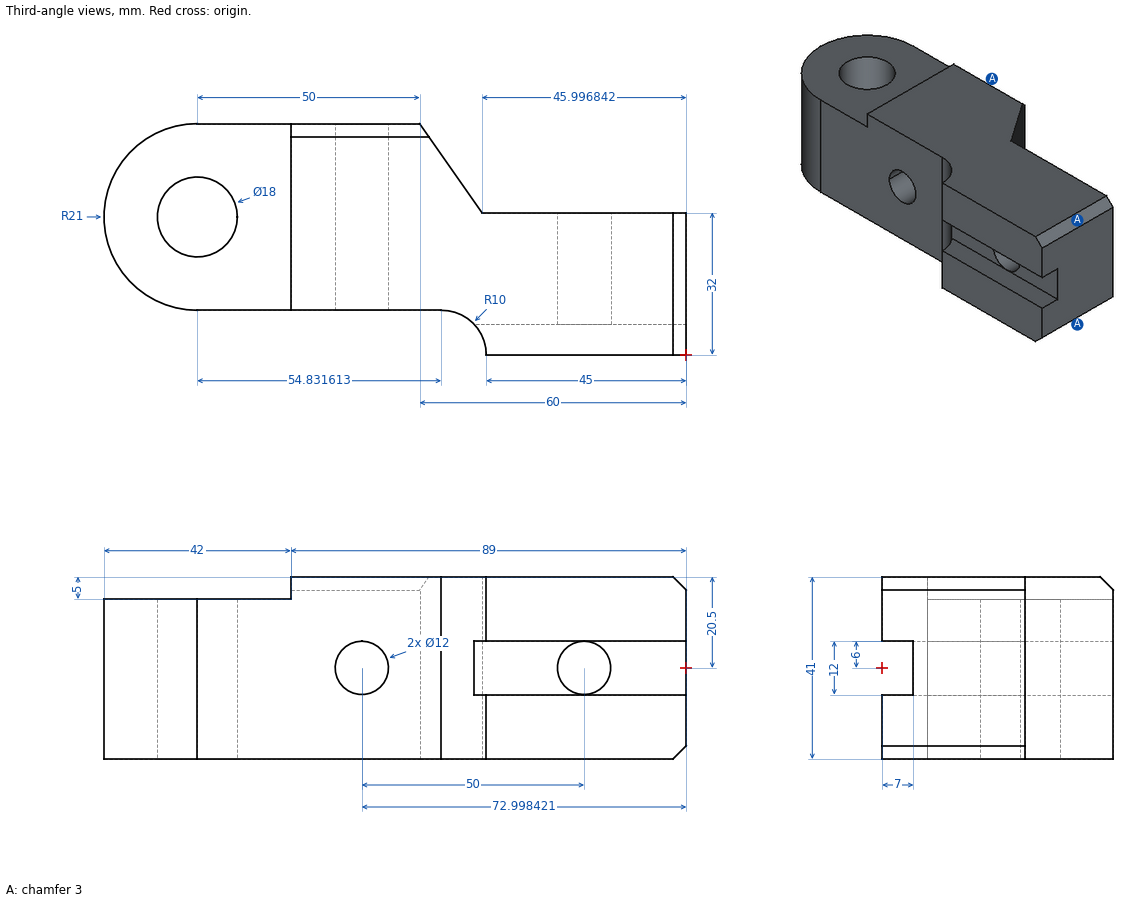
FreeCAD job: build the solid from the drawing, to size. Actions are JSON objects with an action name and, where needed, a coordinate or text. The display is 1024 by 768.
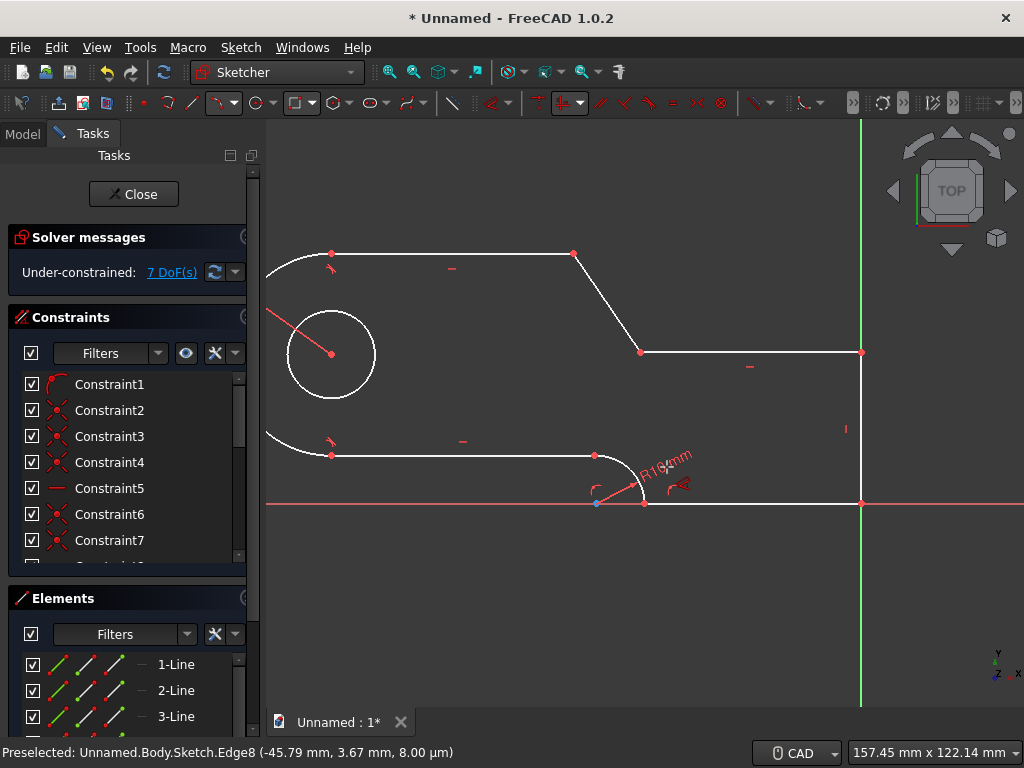
{"action": "left_click", "coordinate": [362, 324]}
{"action": "left_click", "coordinate": [385, 301]}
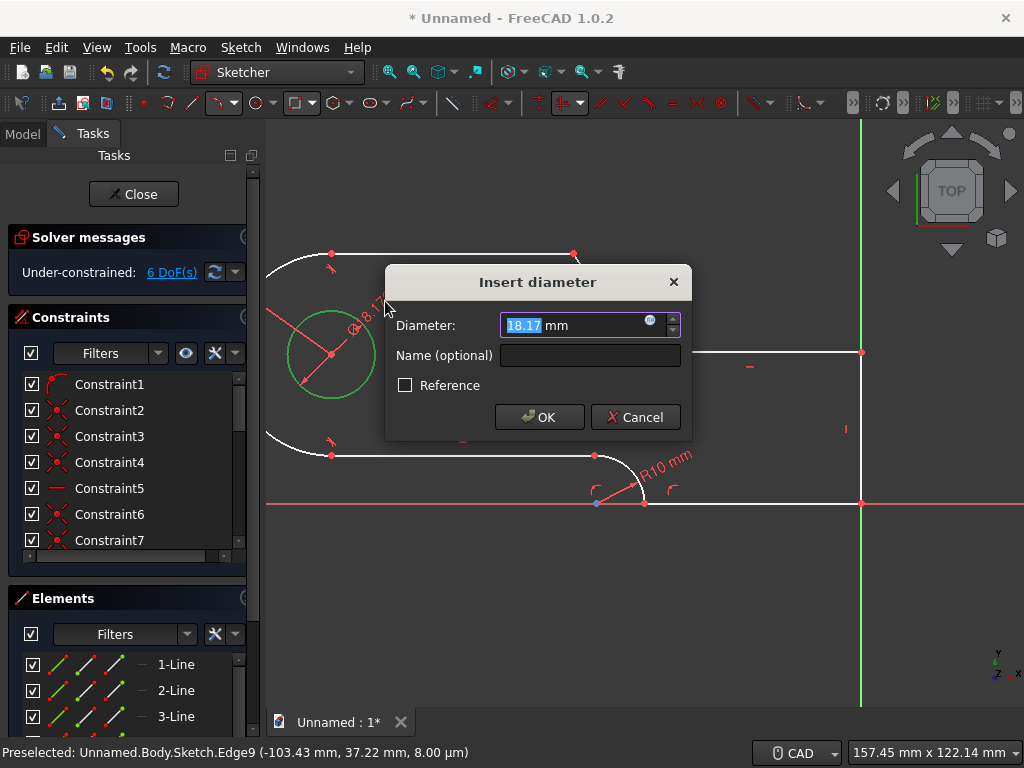
{"action": "type", "text": "18"}
{"action": "key", "text": "Return"}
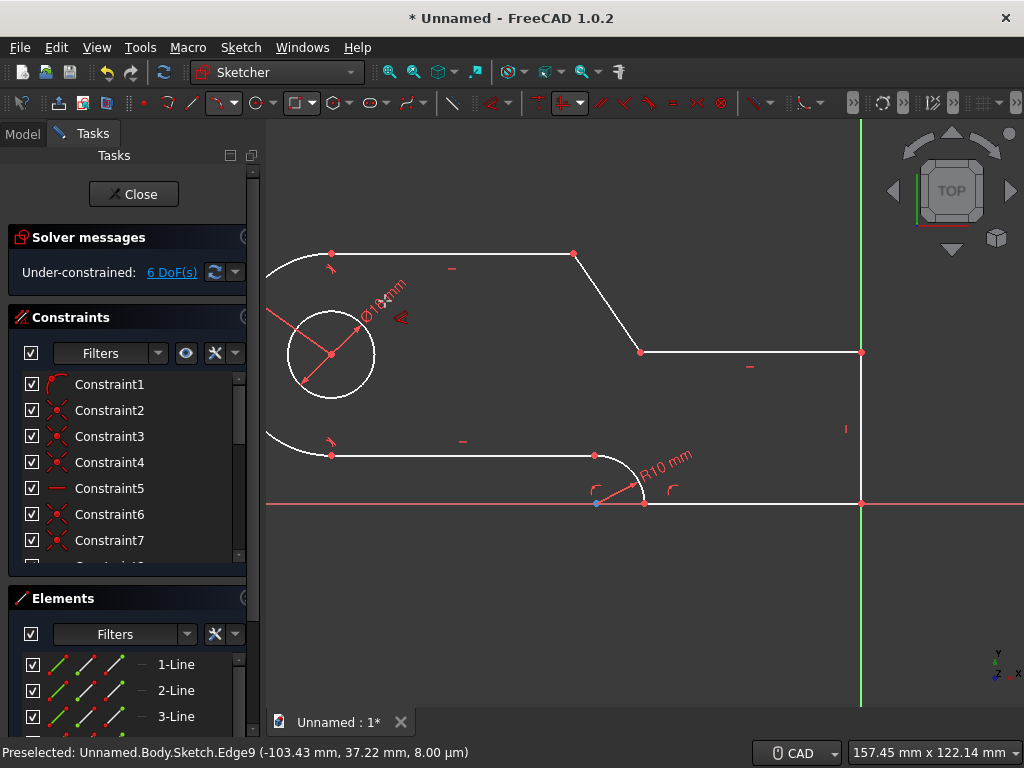
{"action": "left_click", "coordinate": [709, 504]}
{"action": "left_click", "coordinate": [752, 538]}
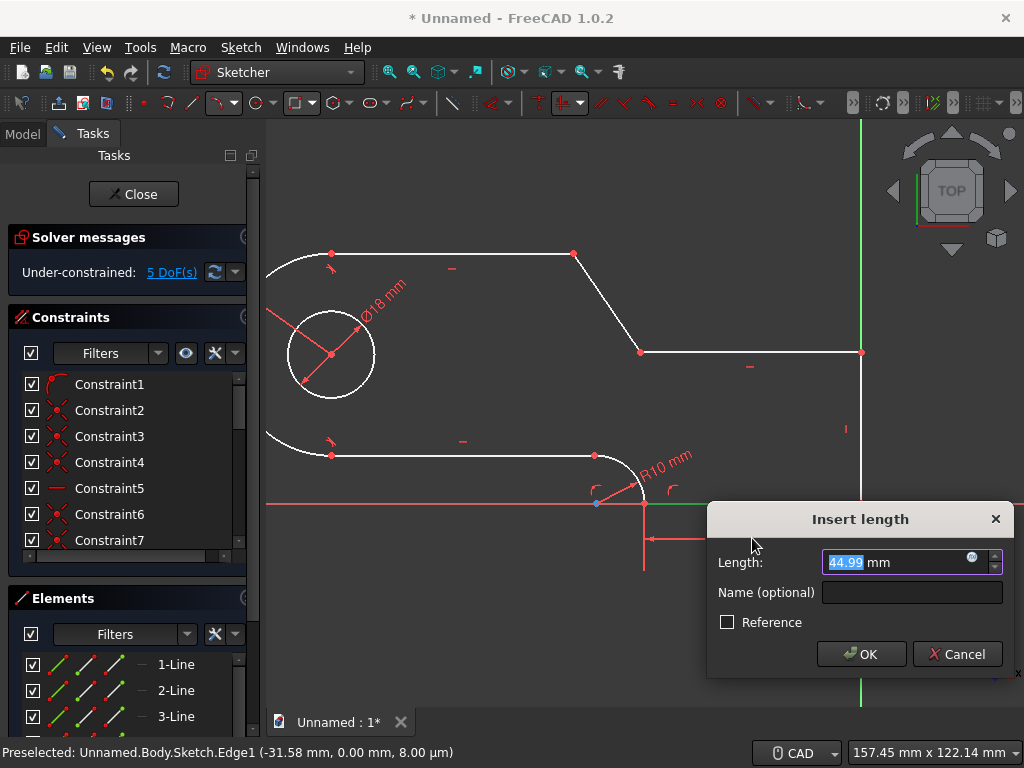
{"action": "type", "text": "45"}
{"action": "key", "text": "Return"}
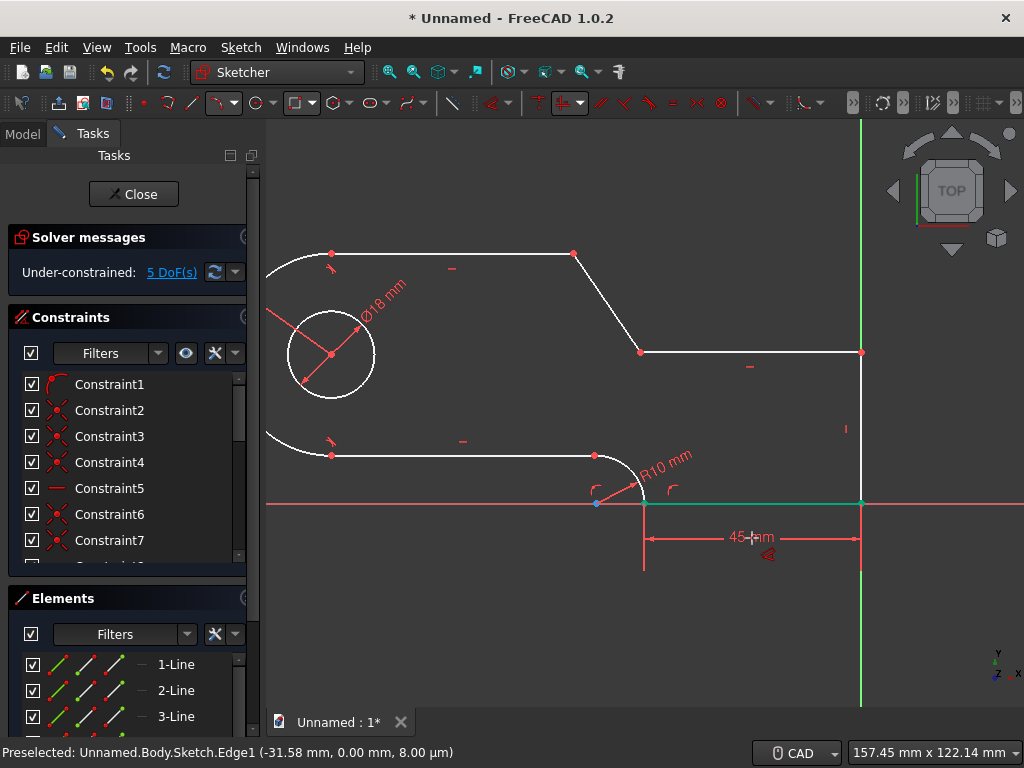
{"action": "scroll", "coordinate": [639, 483], "scroll_direction": "down", "scroll_amount": 2}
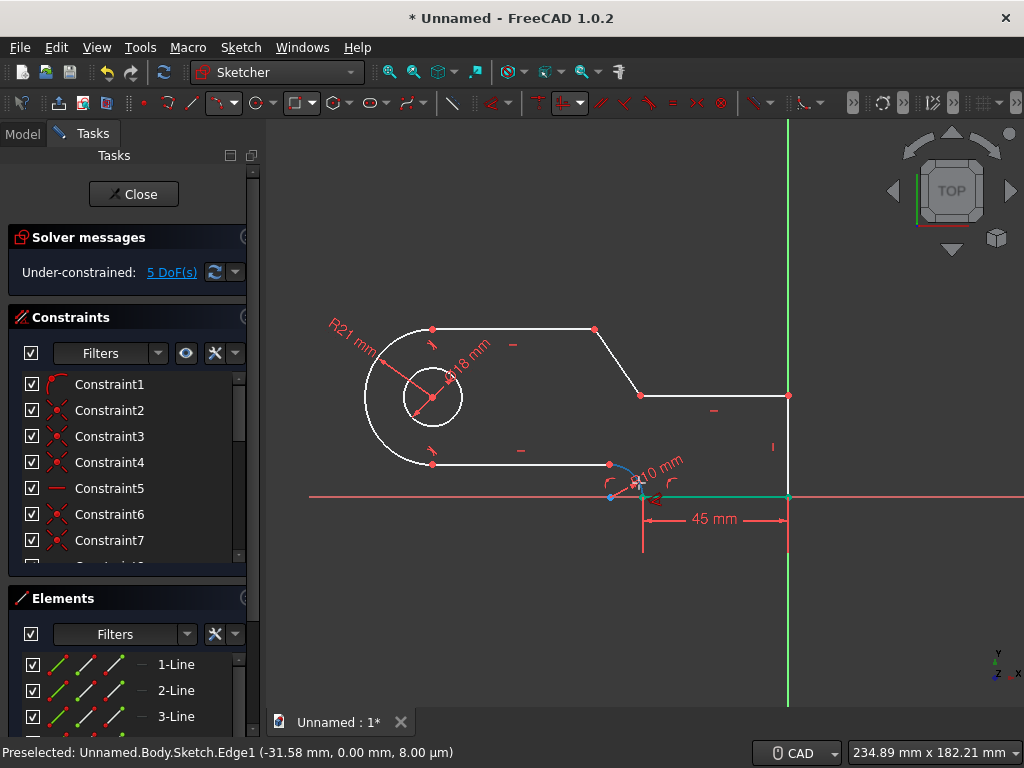
{"action": "left_click", "coordinate": [788, 467]}
{"action": "left_click", "coordinate": [822, 446]}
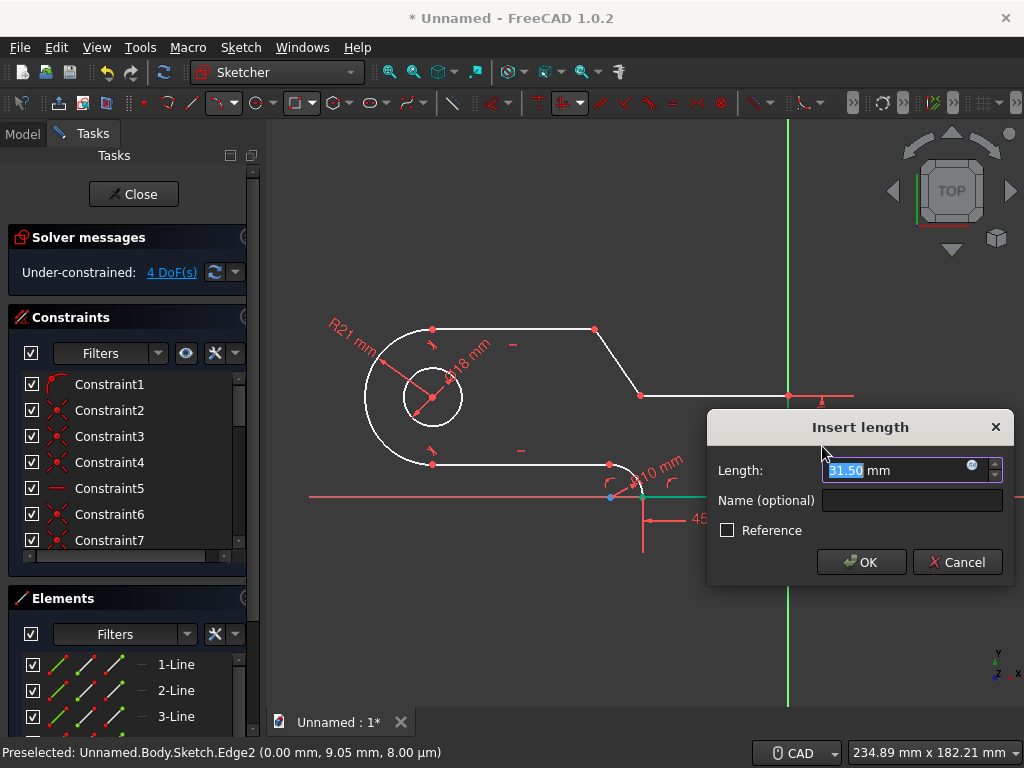
{"action": "type", "text": "32"}
{"action": "key", "text": "Return"}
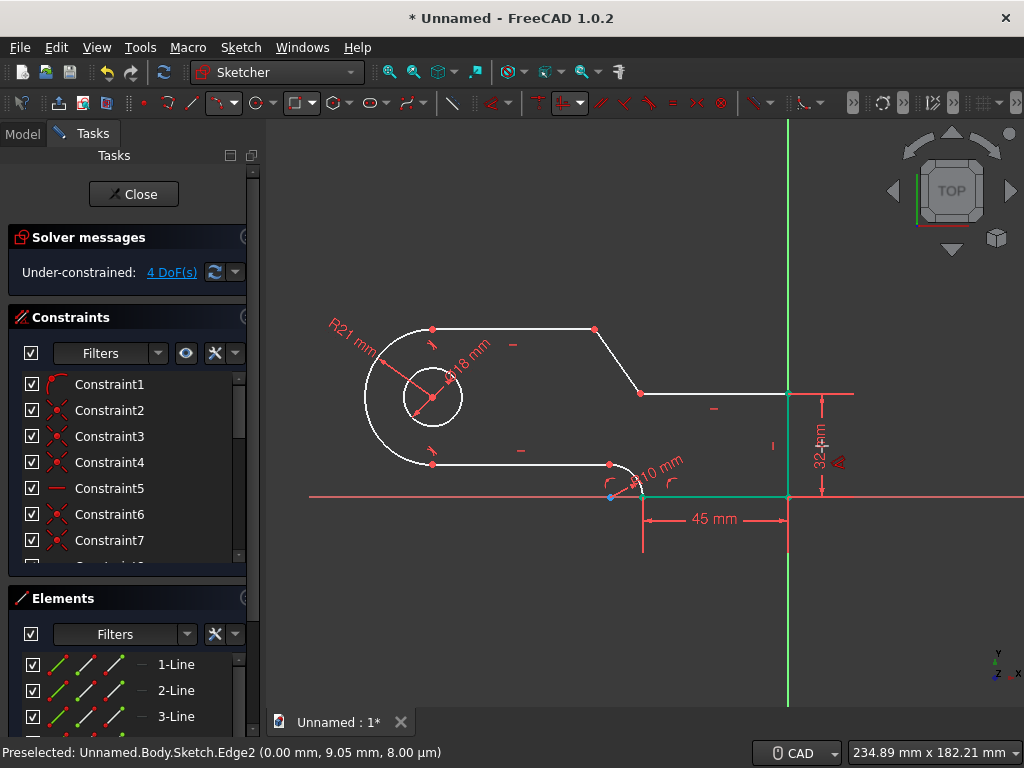
{"action": "left_click", "coordinate": [546, 329]}
{"action": "left_click", "coordinate": [514, 295]}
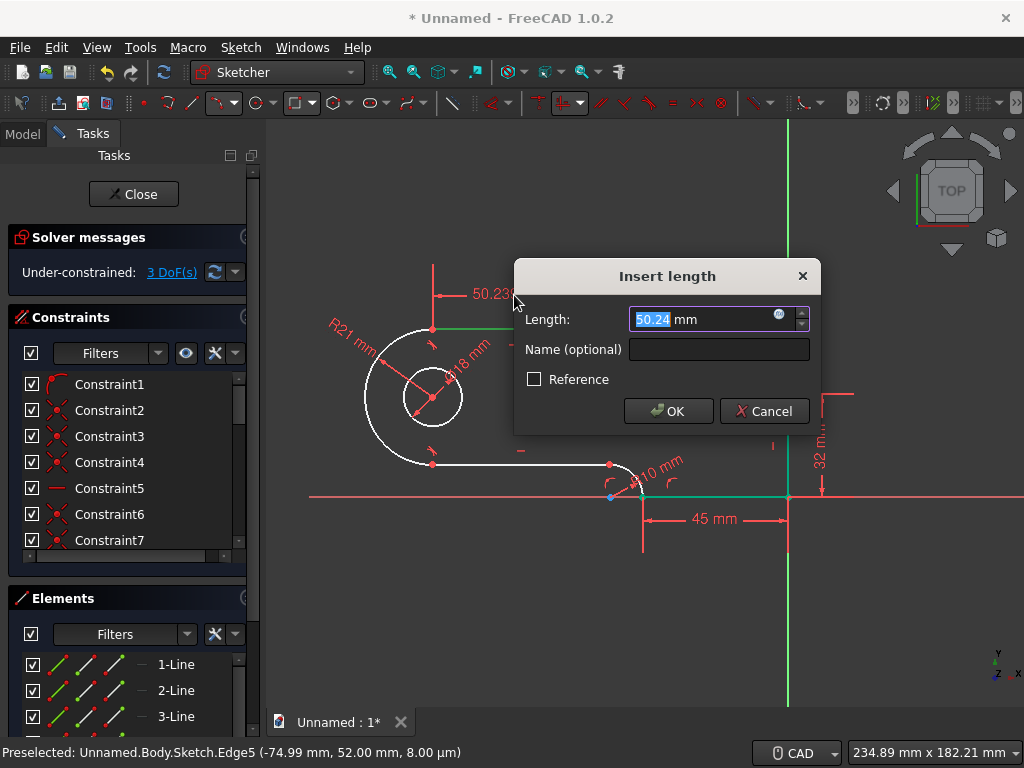
{"action": "type", "text": "50"}
{"action": "key", "text": "Return"}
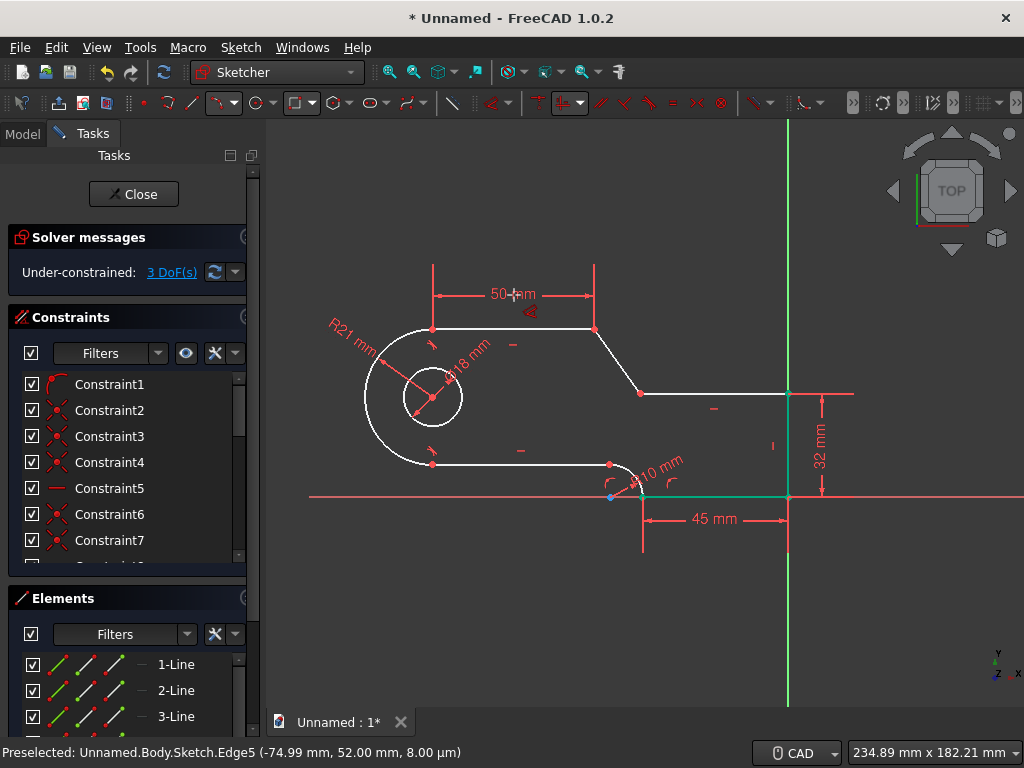
{"action": "left_click", "coordinate": [594, 329]}
{"action": "left_click", "coordinate": [623, 531]}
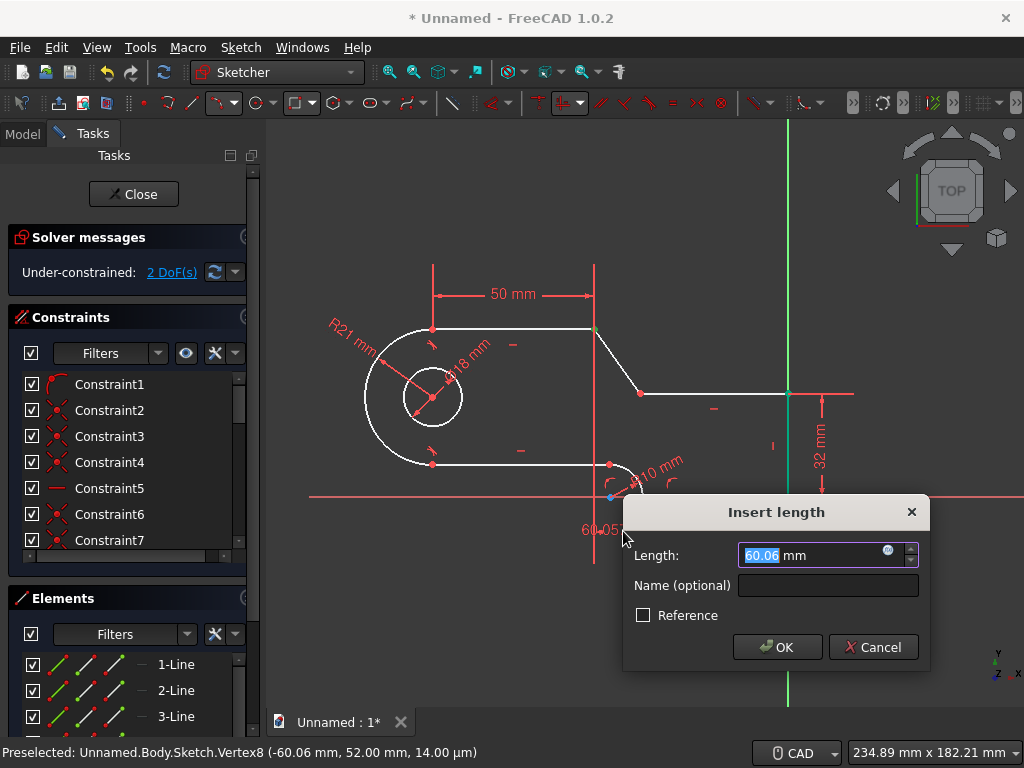
{"action": "type", "text": "60"}
{"action": "key", "text": "Return"}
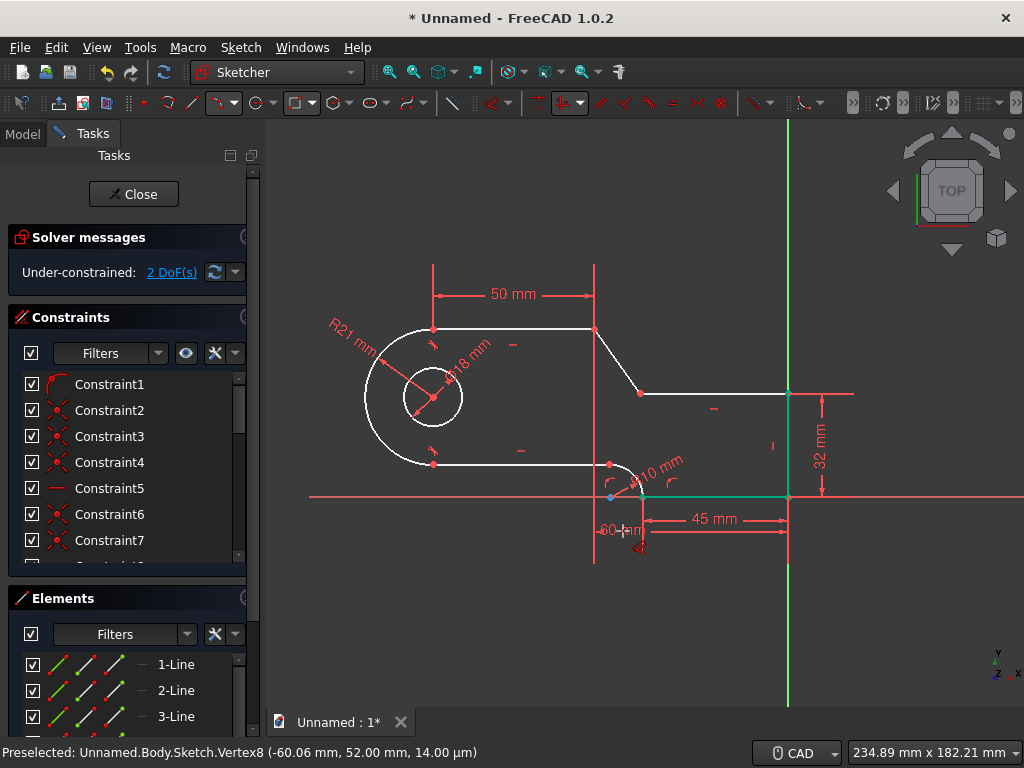
{"action": "left_click", "coordinate": [744, 394]}
{"action": "left_click", "coordinate": [714, 360]}